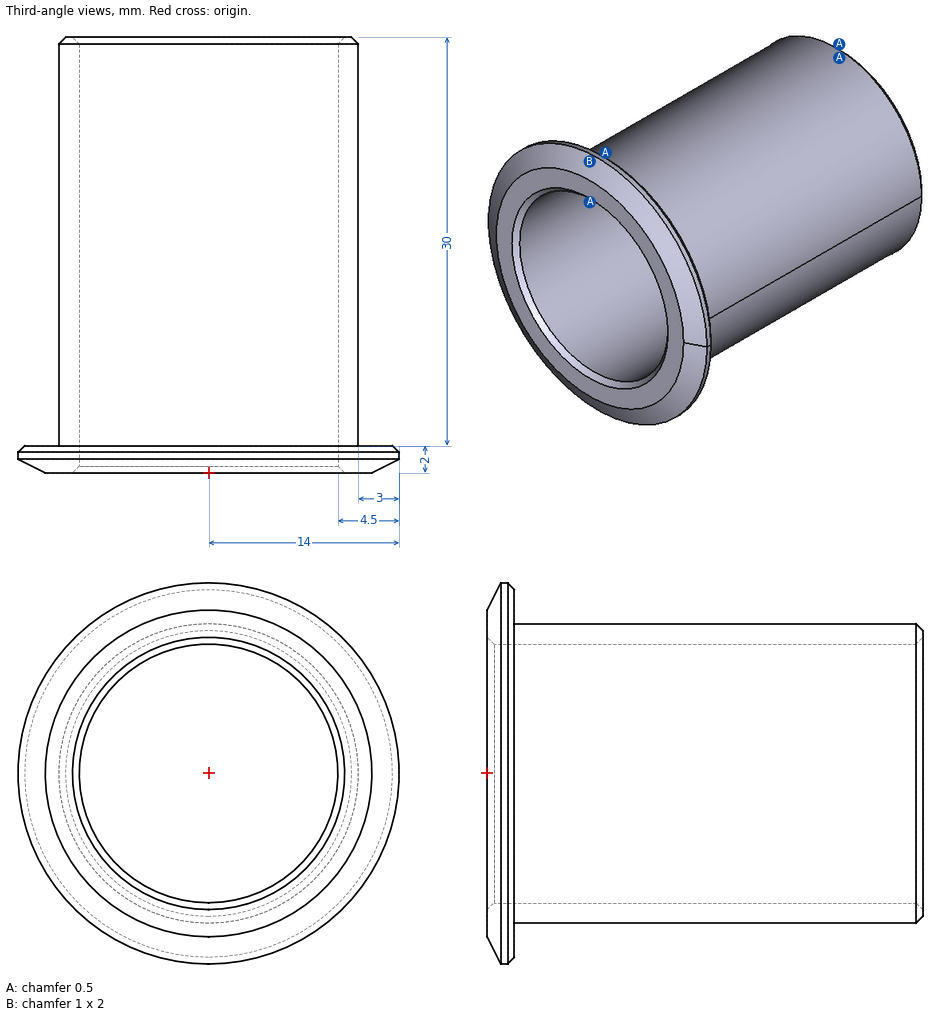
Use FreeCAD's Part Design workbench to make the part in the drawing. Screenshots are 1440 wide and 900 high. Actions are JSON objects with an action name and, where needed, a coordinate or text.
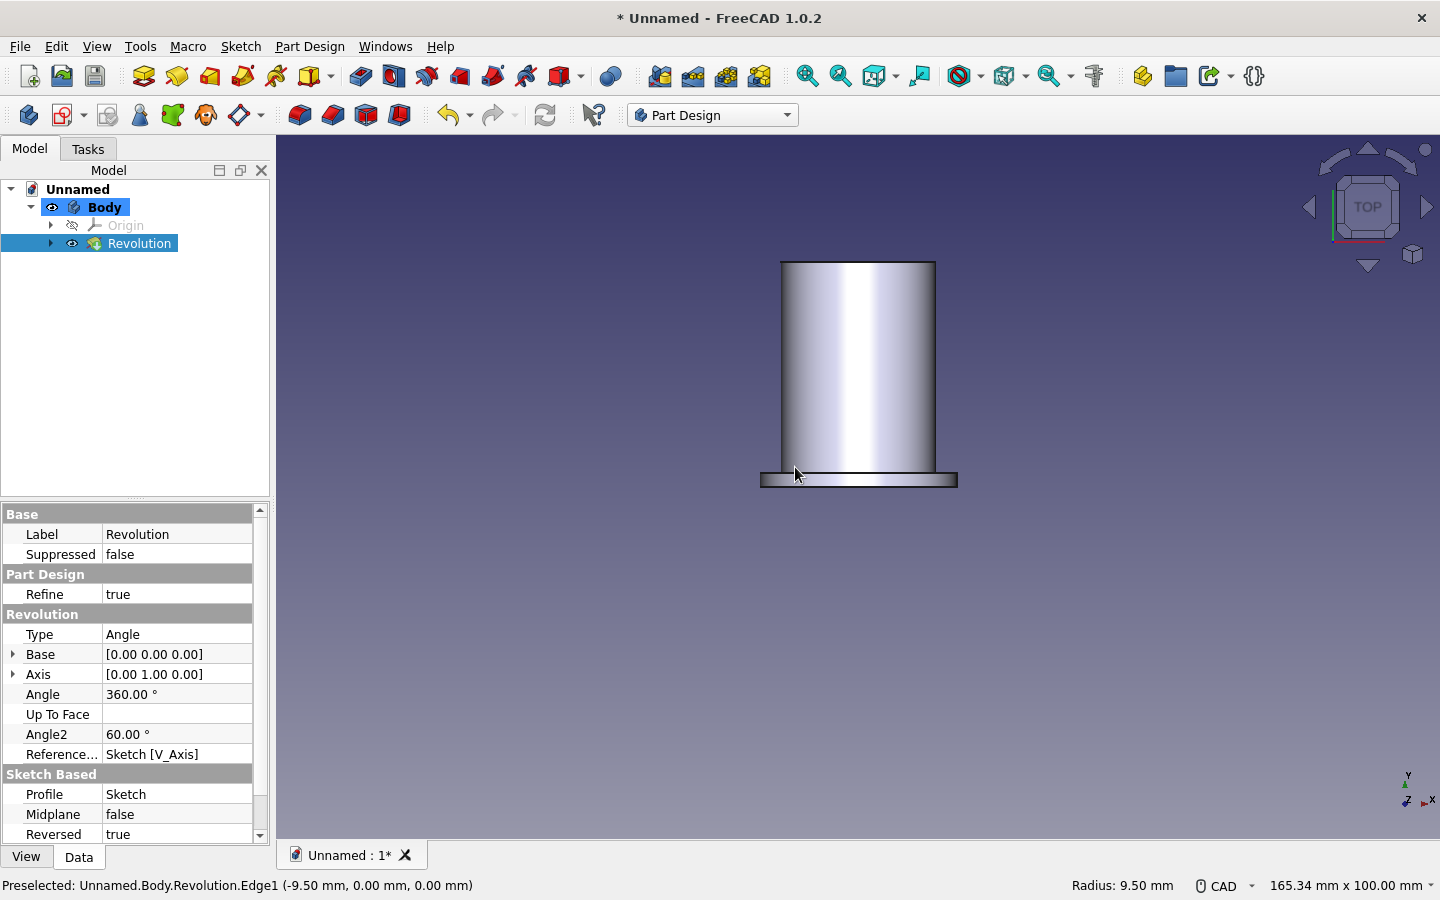
{"action": "left_click", "coordinate": [808, 76]}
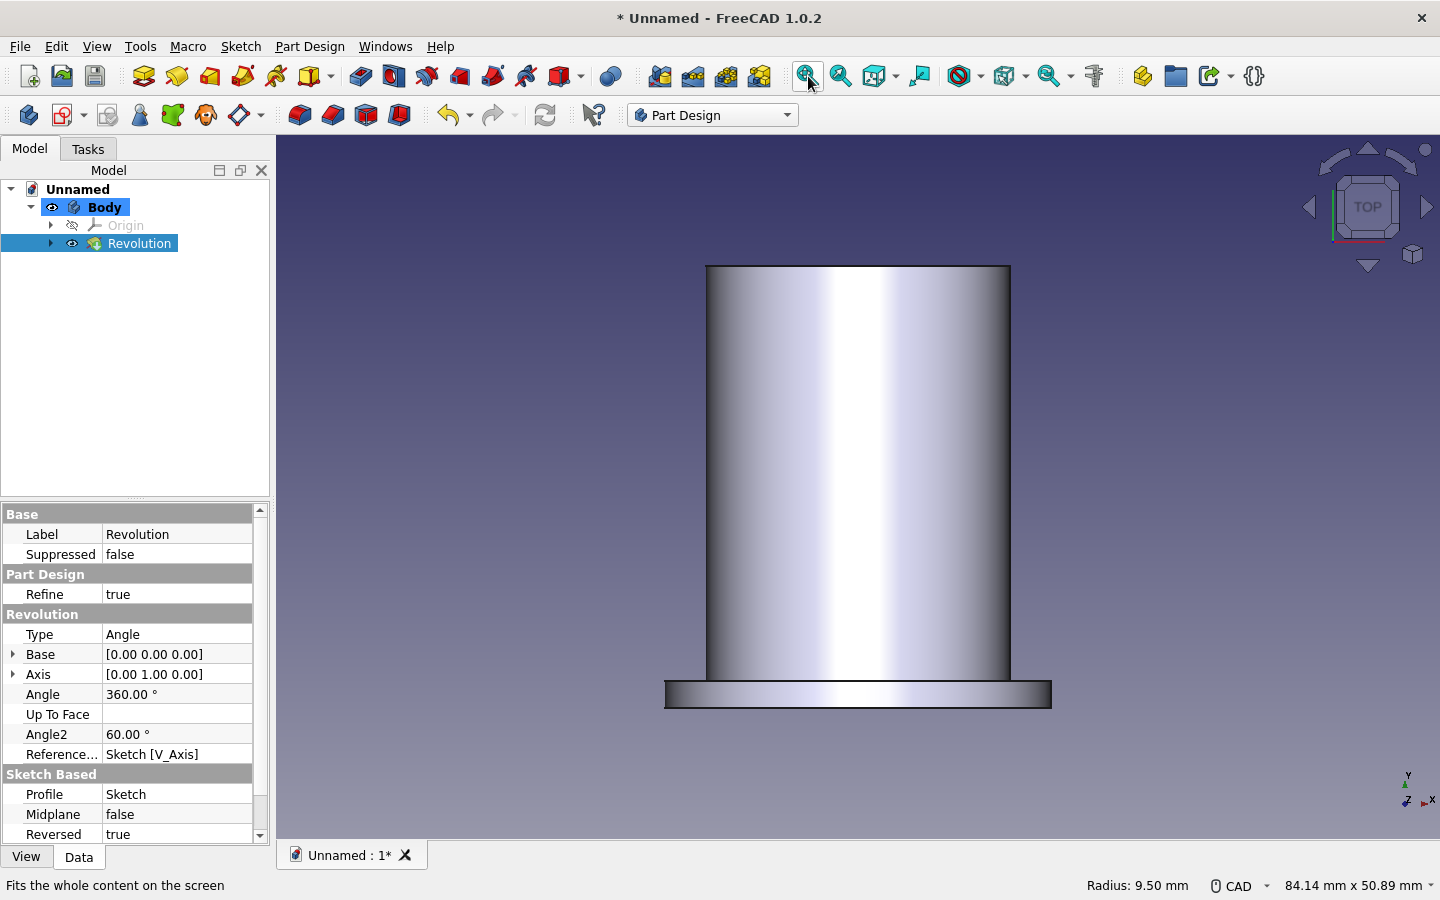
{"action": "left_click", "coordinate": [735, 265], "text": "ctrl"}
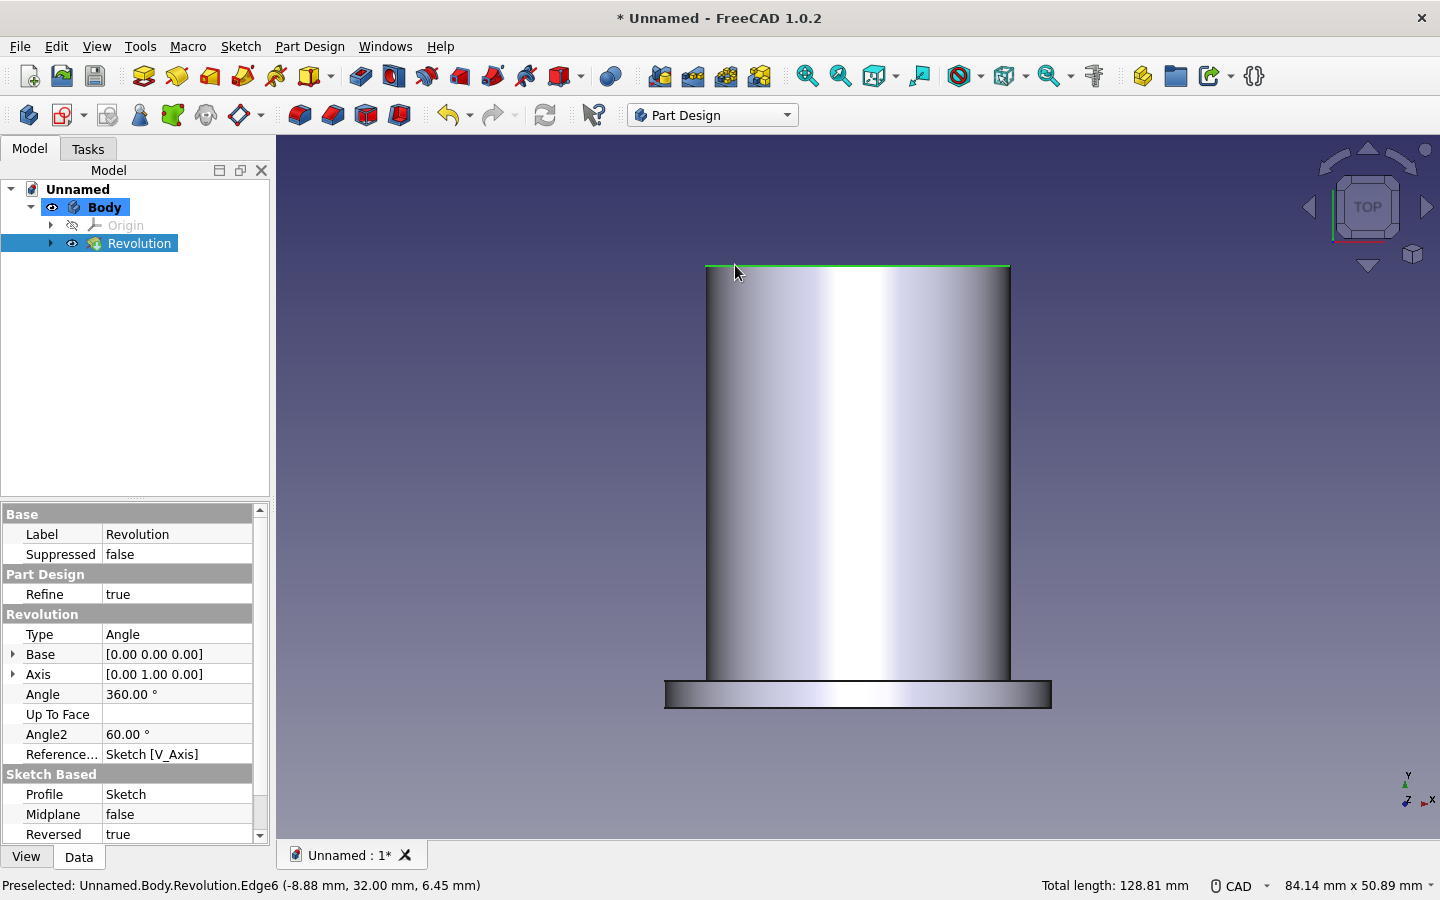
{"action": "left_click", "coordinate": [701, 680], "text": "ctrl"}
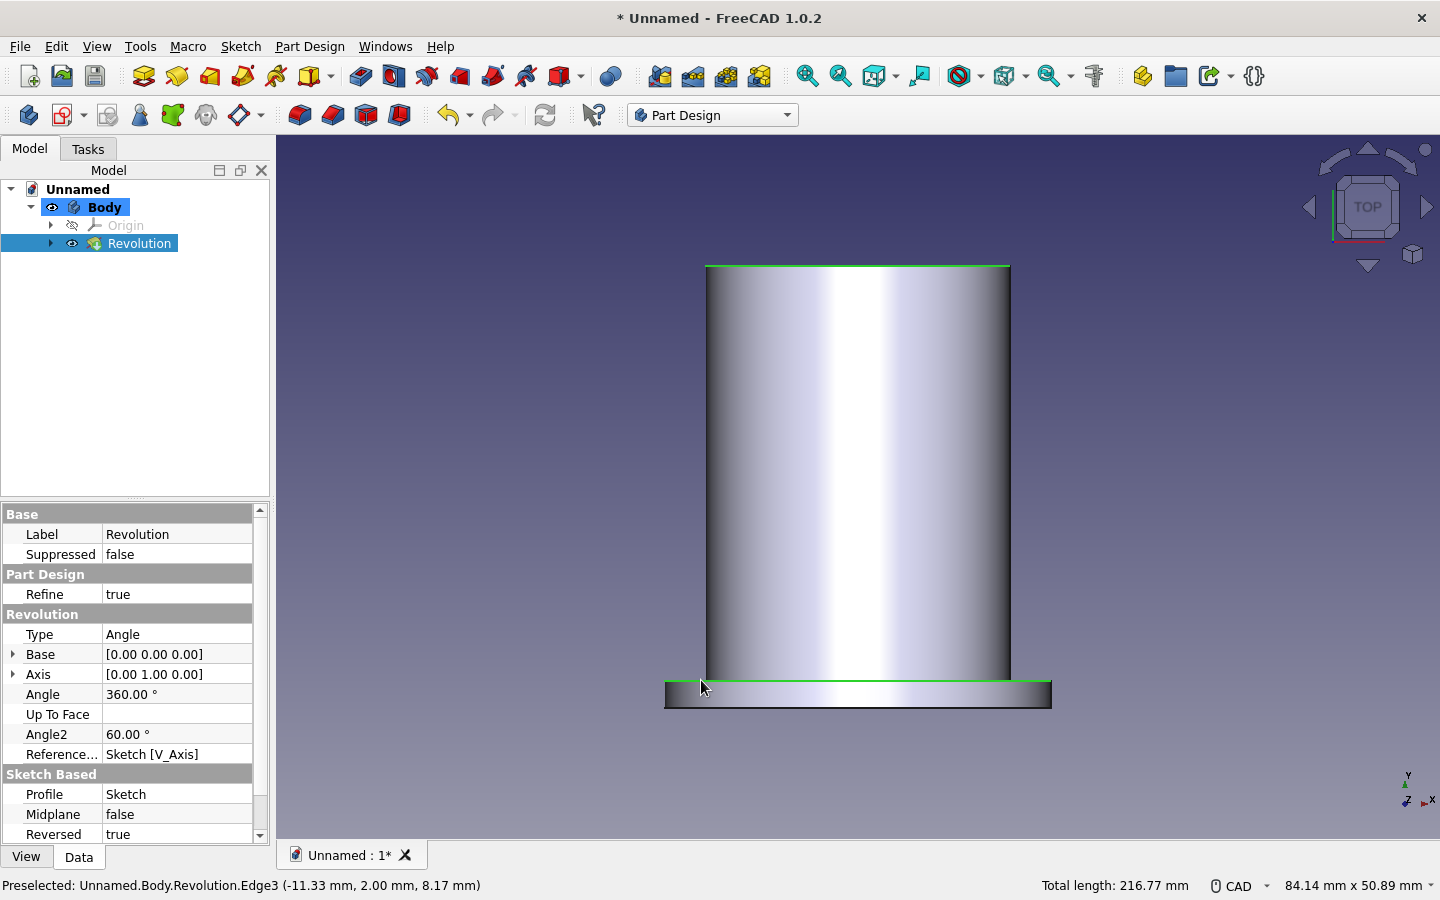
{"action": "key", "text": "1"}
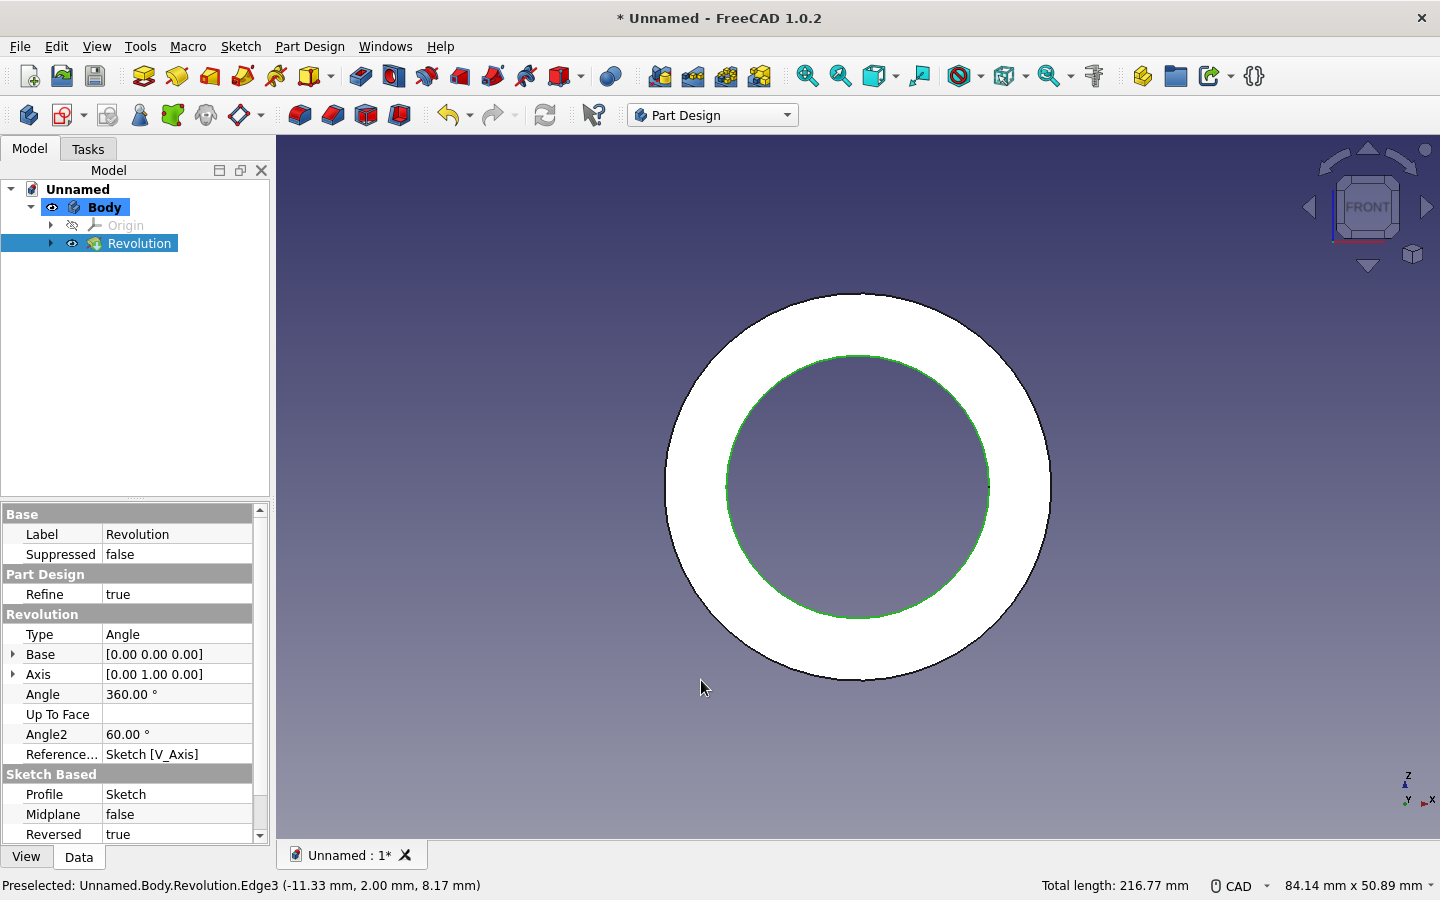
{"action": "key", "text": "3"}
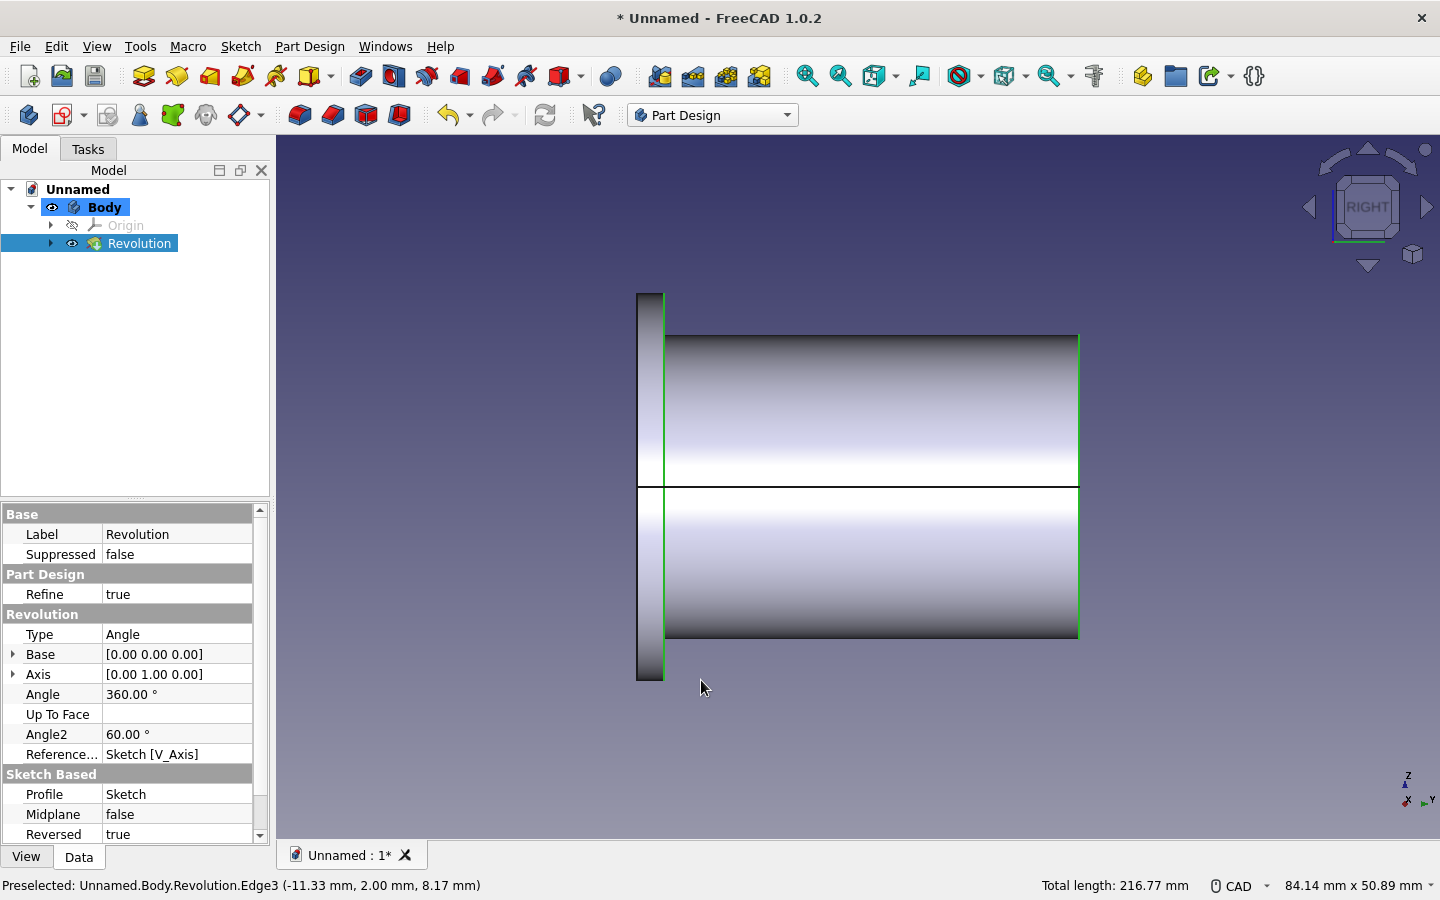
{"action": "key", "text": "5"}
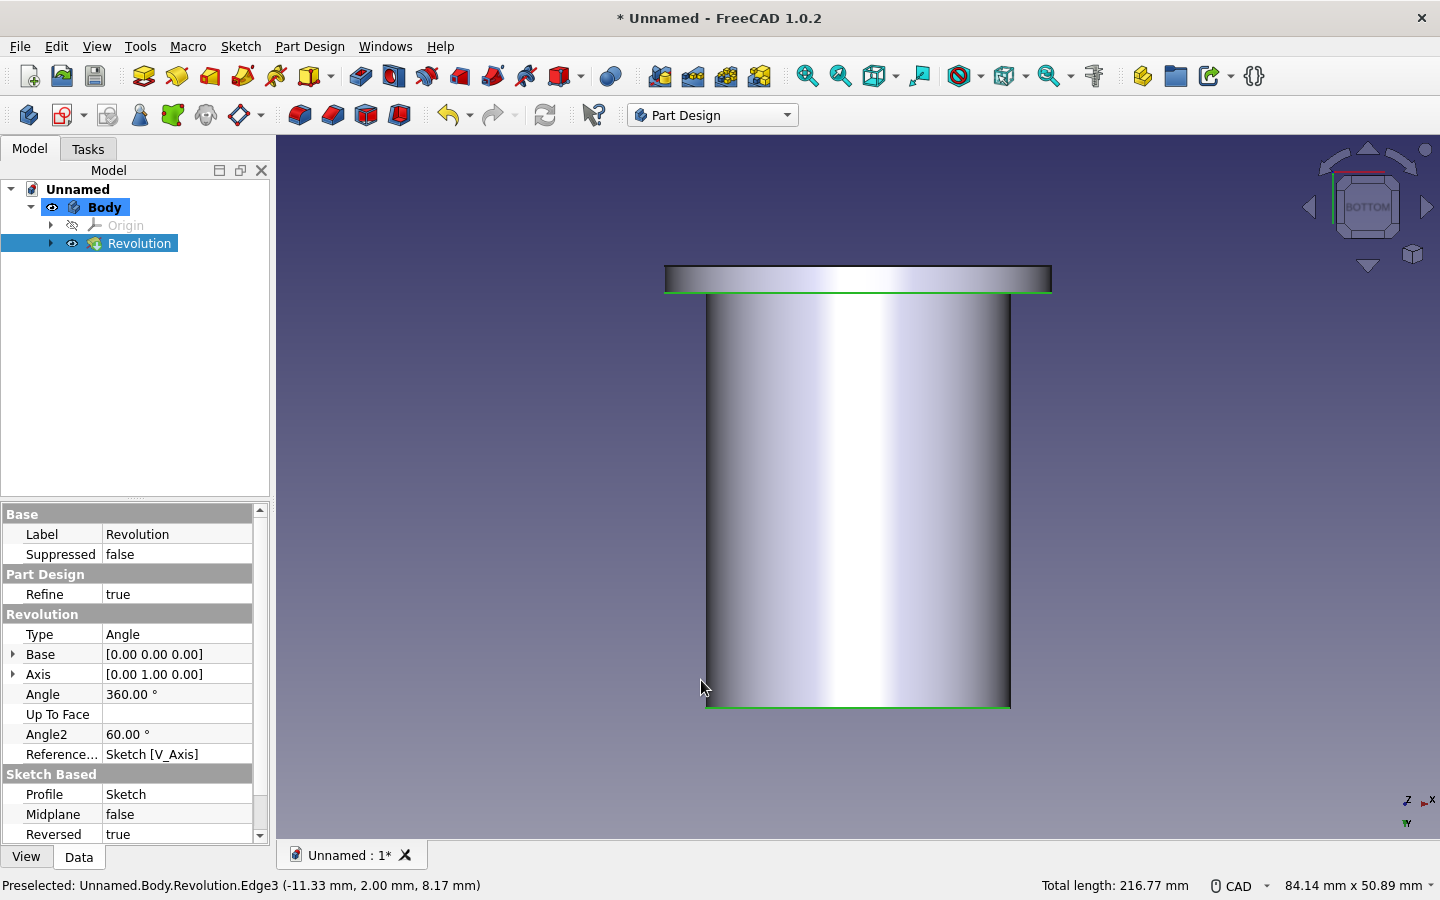
{"action": "key", "text": "4"}